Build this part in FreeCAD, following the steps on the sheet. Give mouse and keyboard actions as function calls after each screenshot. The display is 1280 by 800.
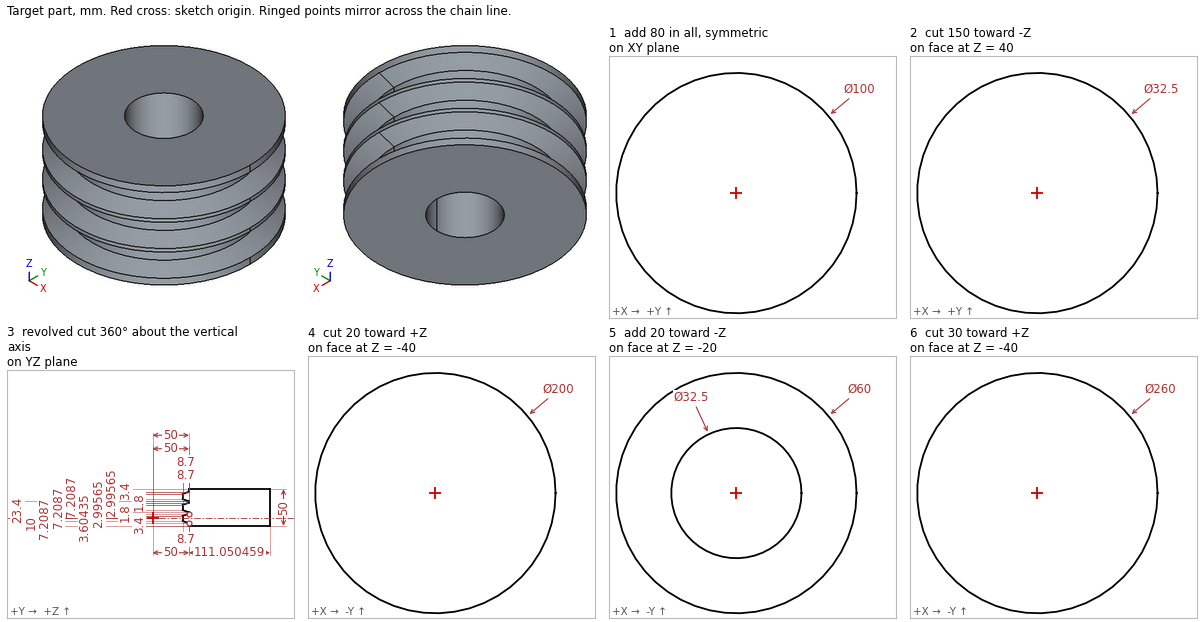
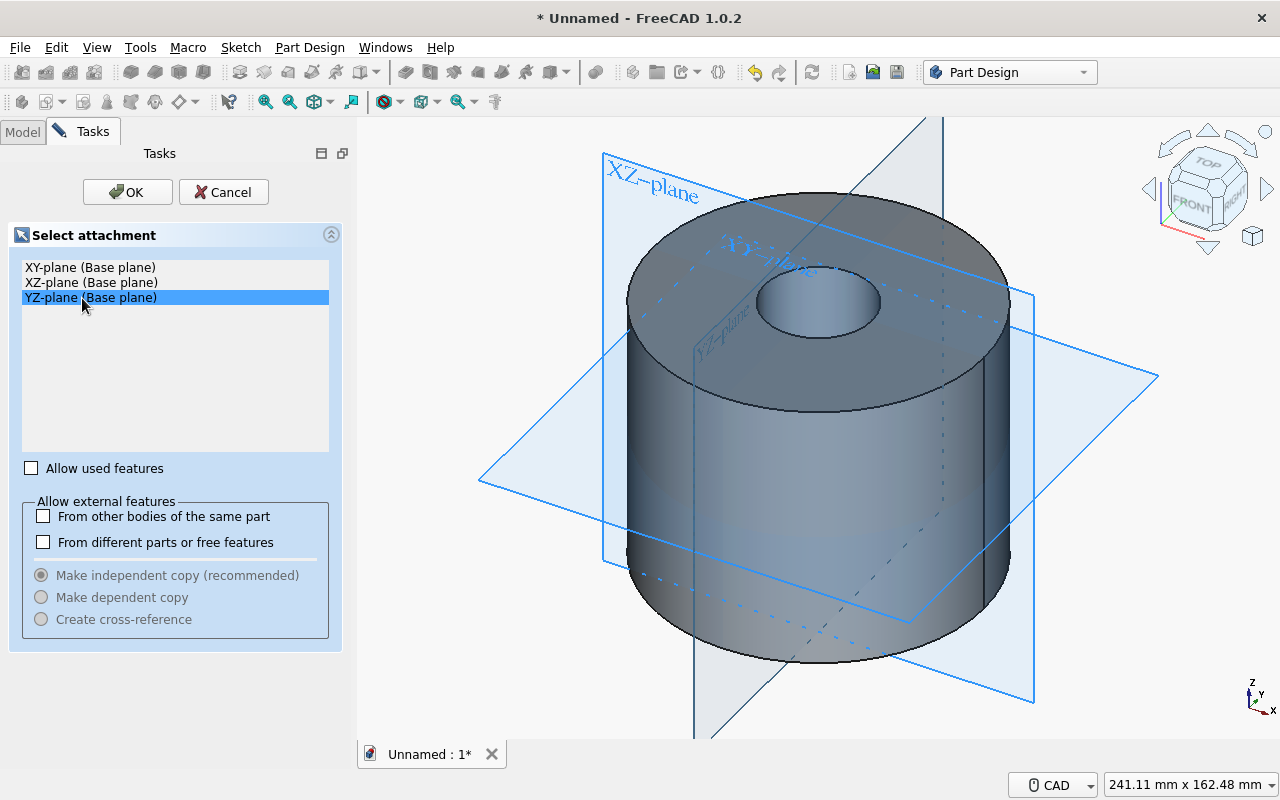
click(128, 192)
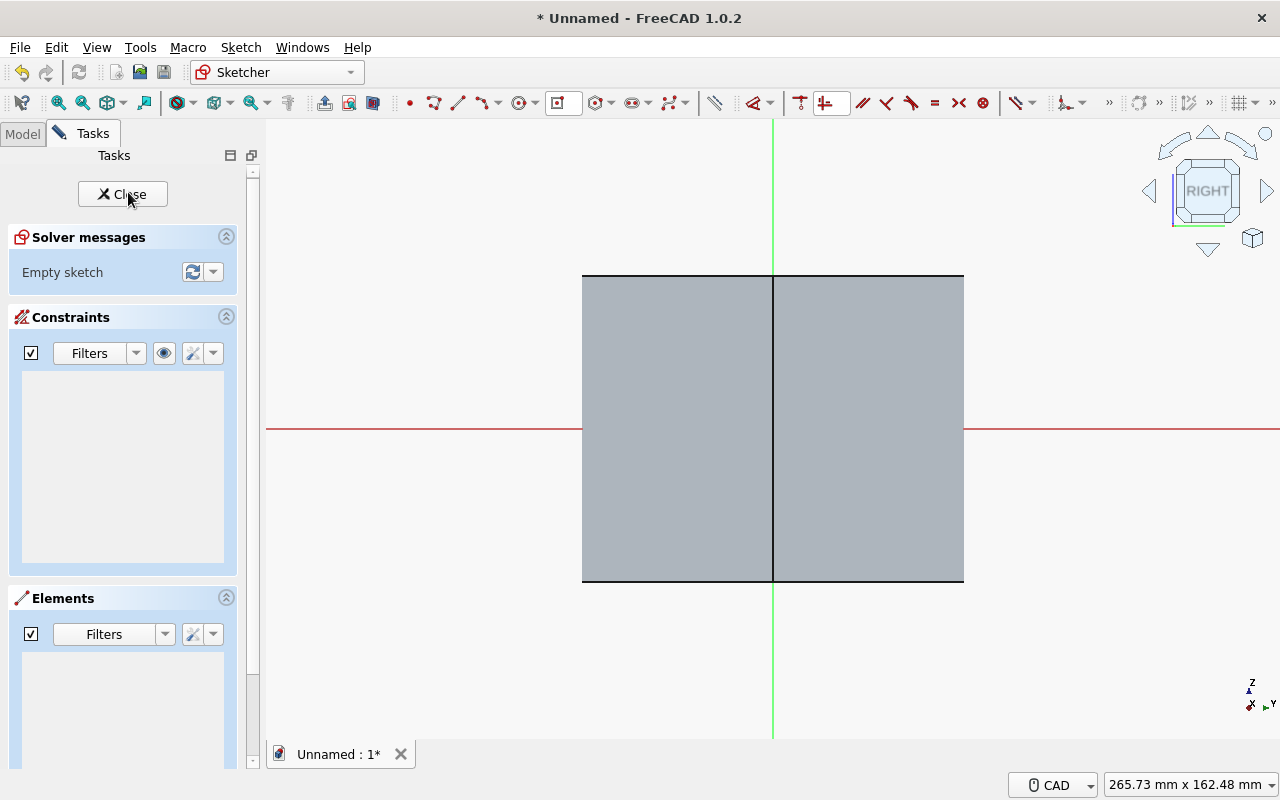
click(374, 104)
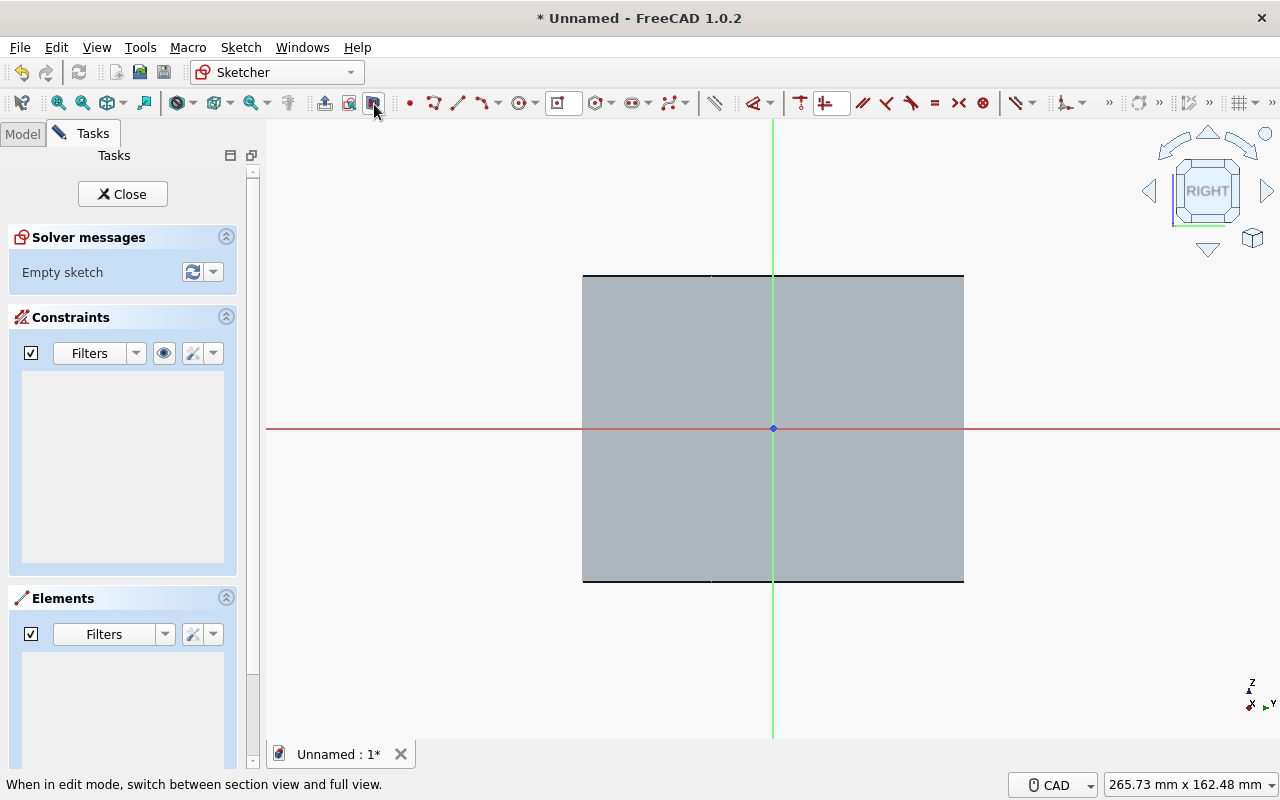
scroll(294, 545, down, 2)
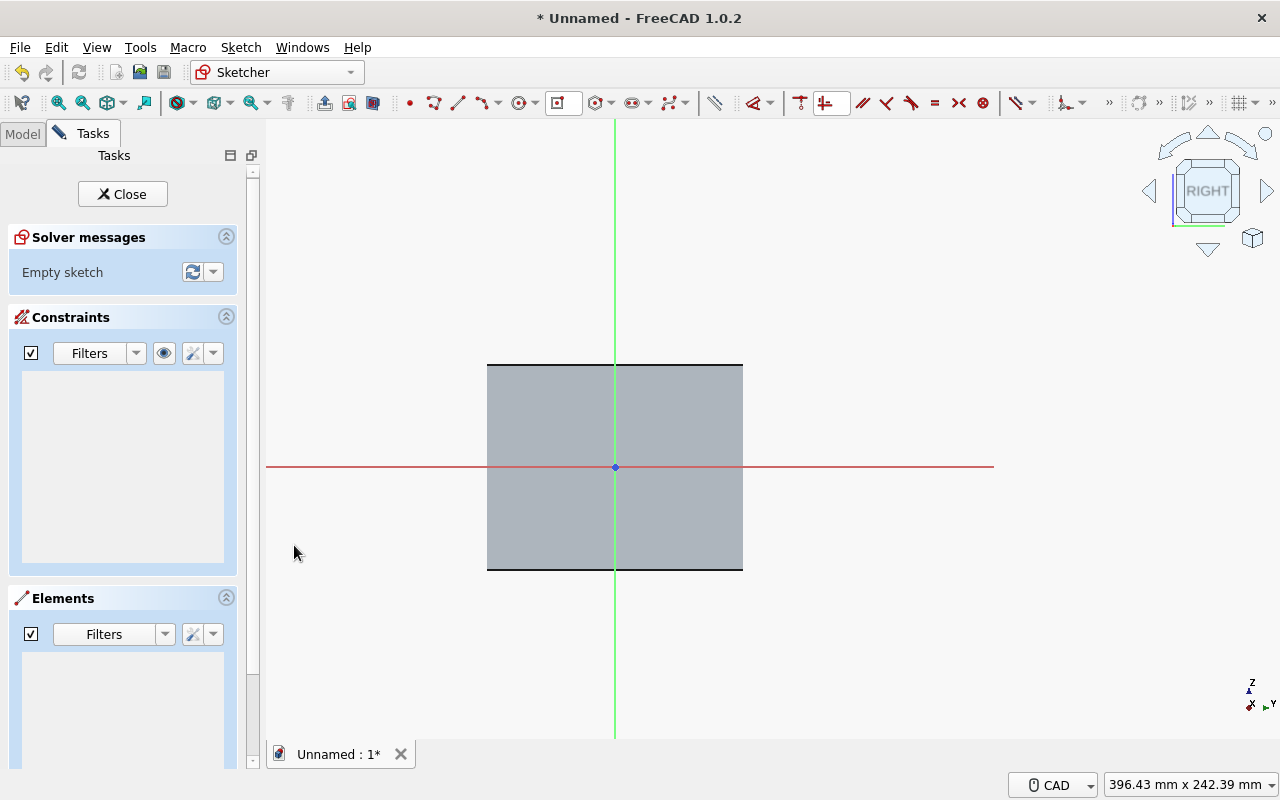
scroll(1058, 429, up, 2)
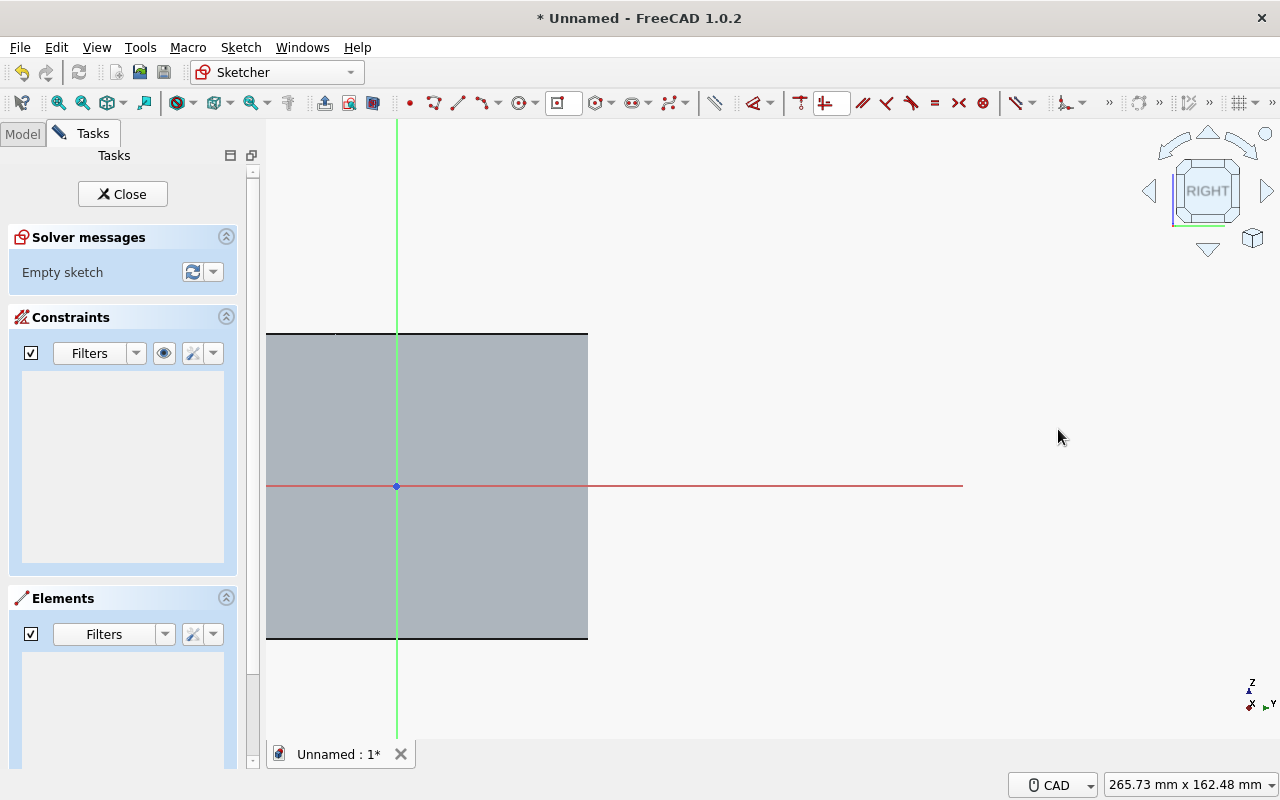
click(434, 104)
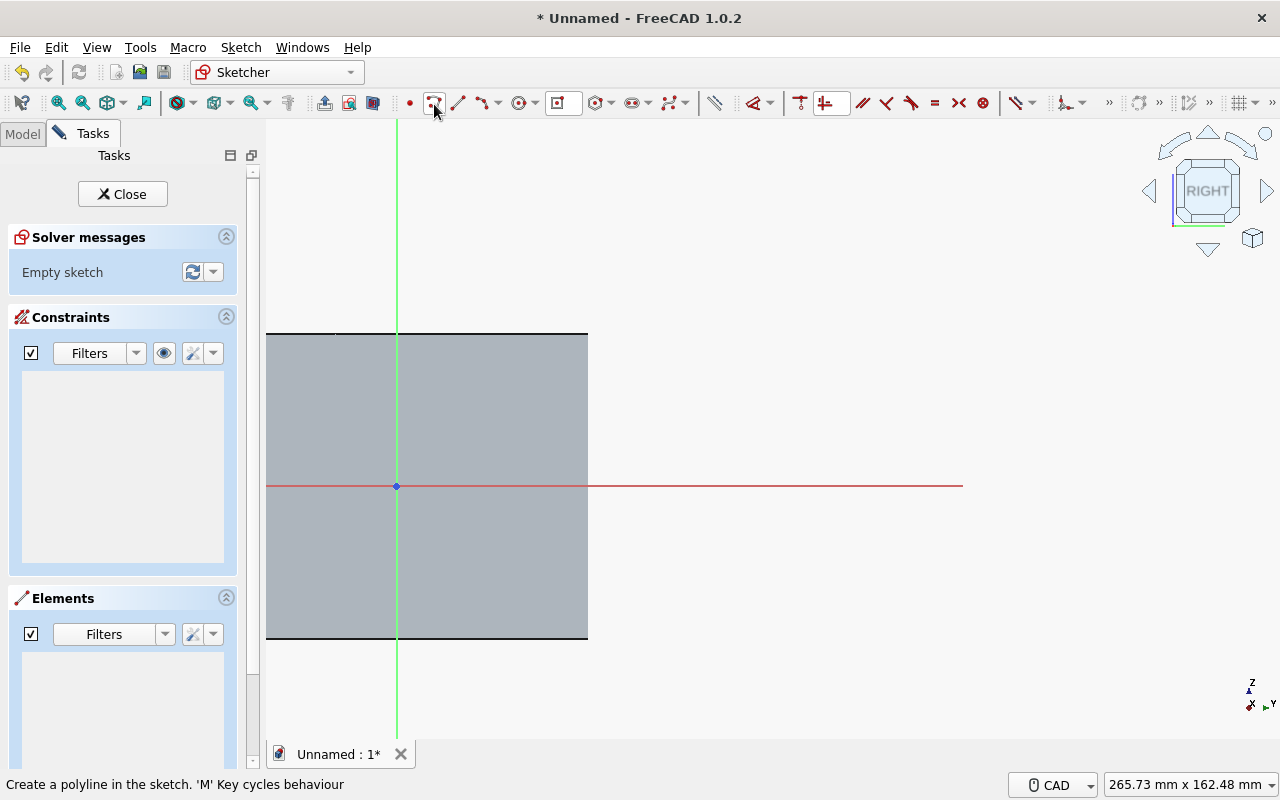
click(554, 472)
click(554, 500)
click(588, 511)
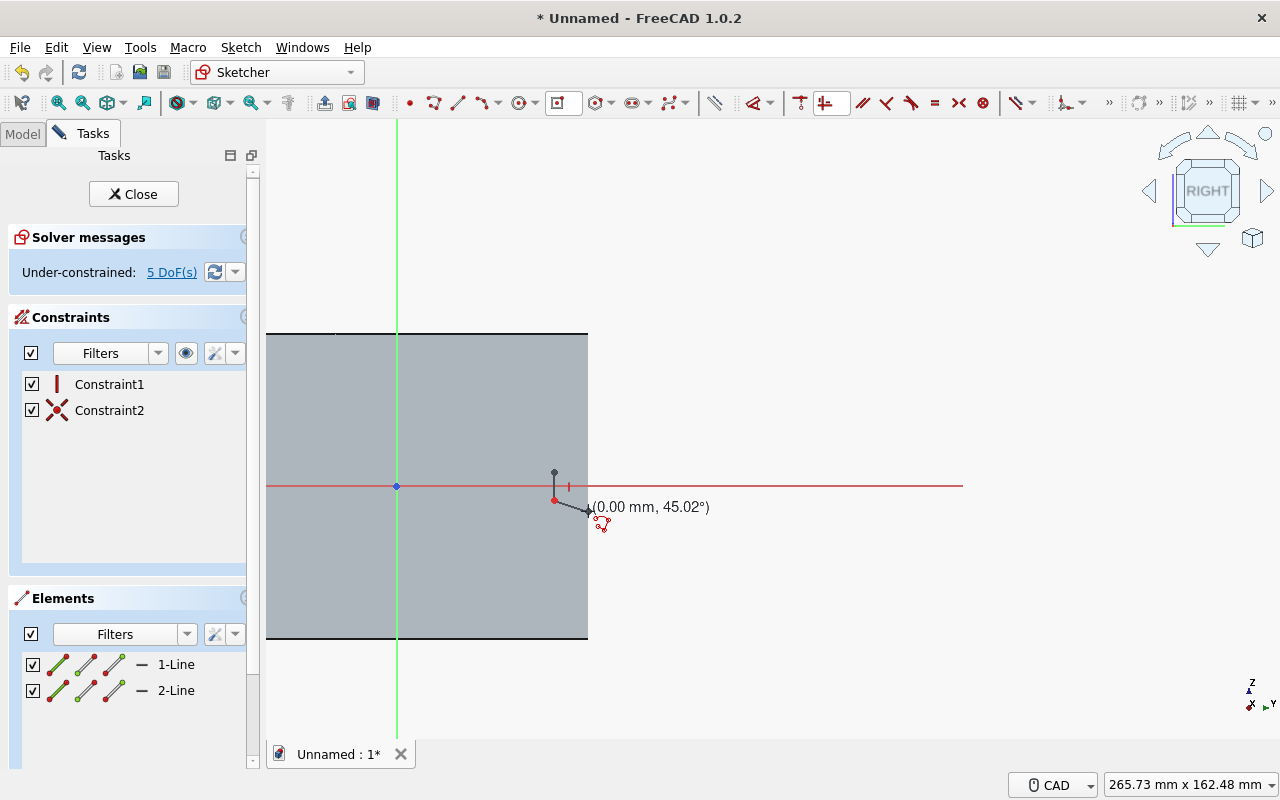
scroll(588, 524, up, 2)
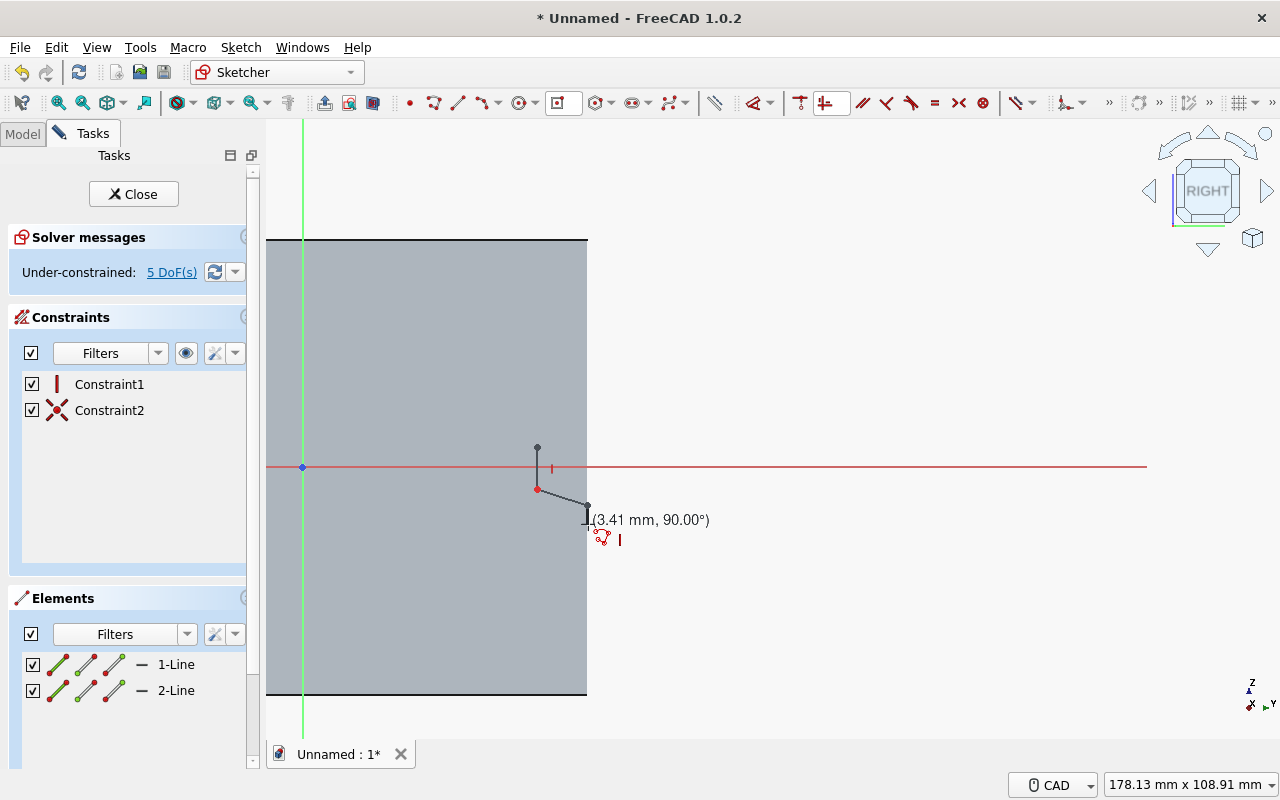
click(588, 524)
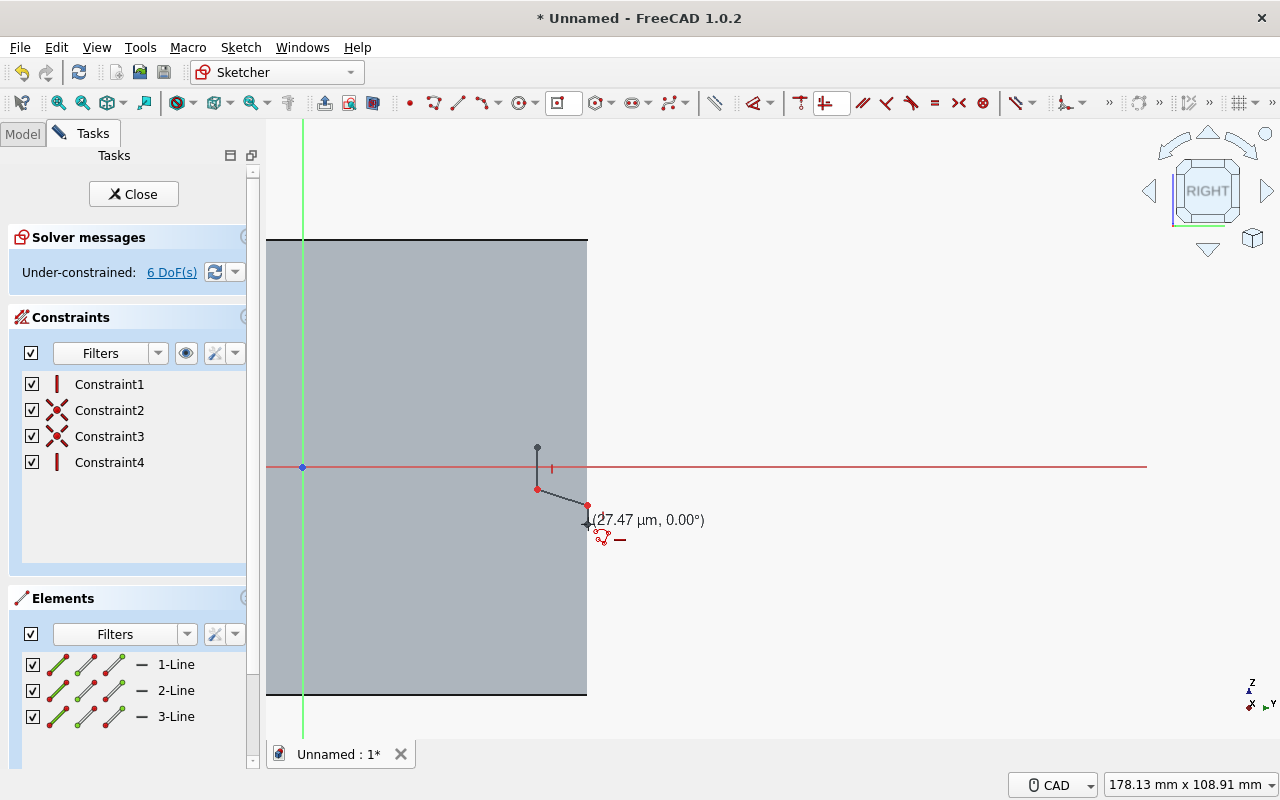
scroll(589, 525, down, 2)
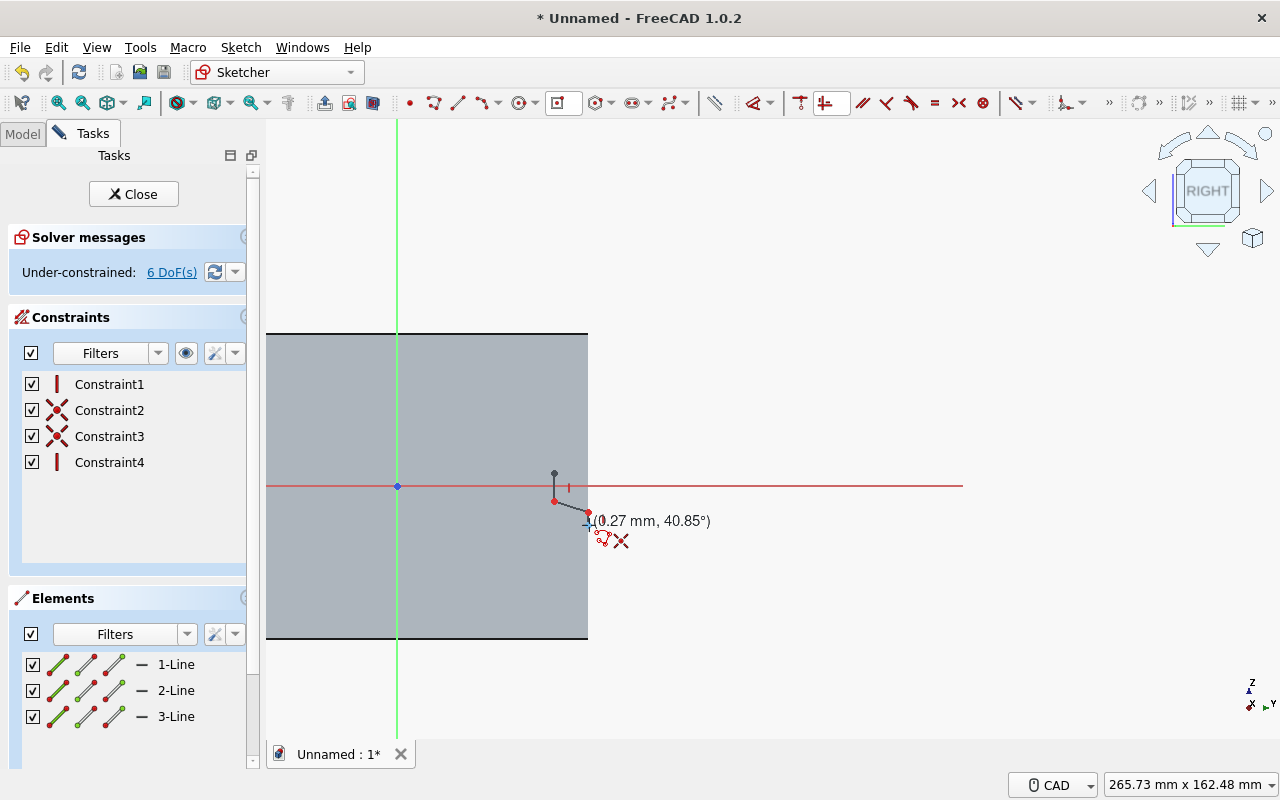
click(1012, 525)
click(1012, 334)
click(588, 334)